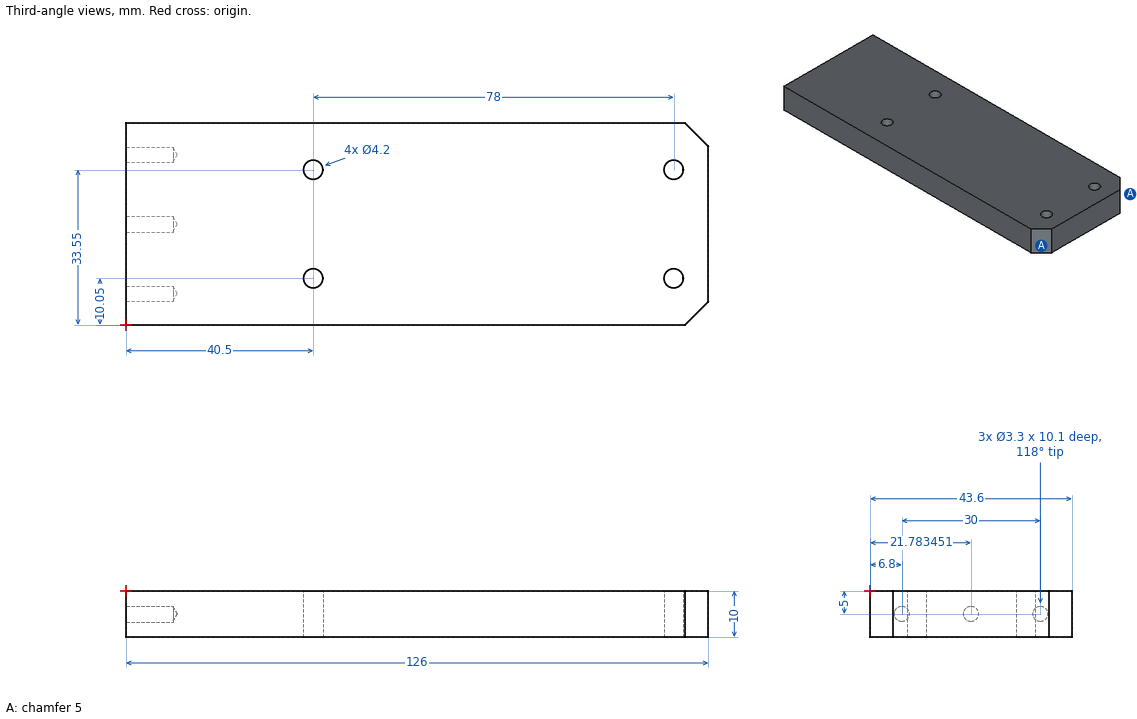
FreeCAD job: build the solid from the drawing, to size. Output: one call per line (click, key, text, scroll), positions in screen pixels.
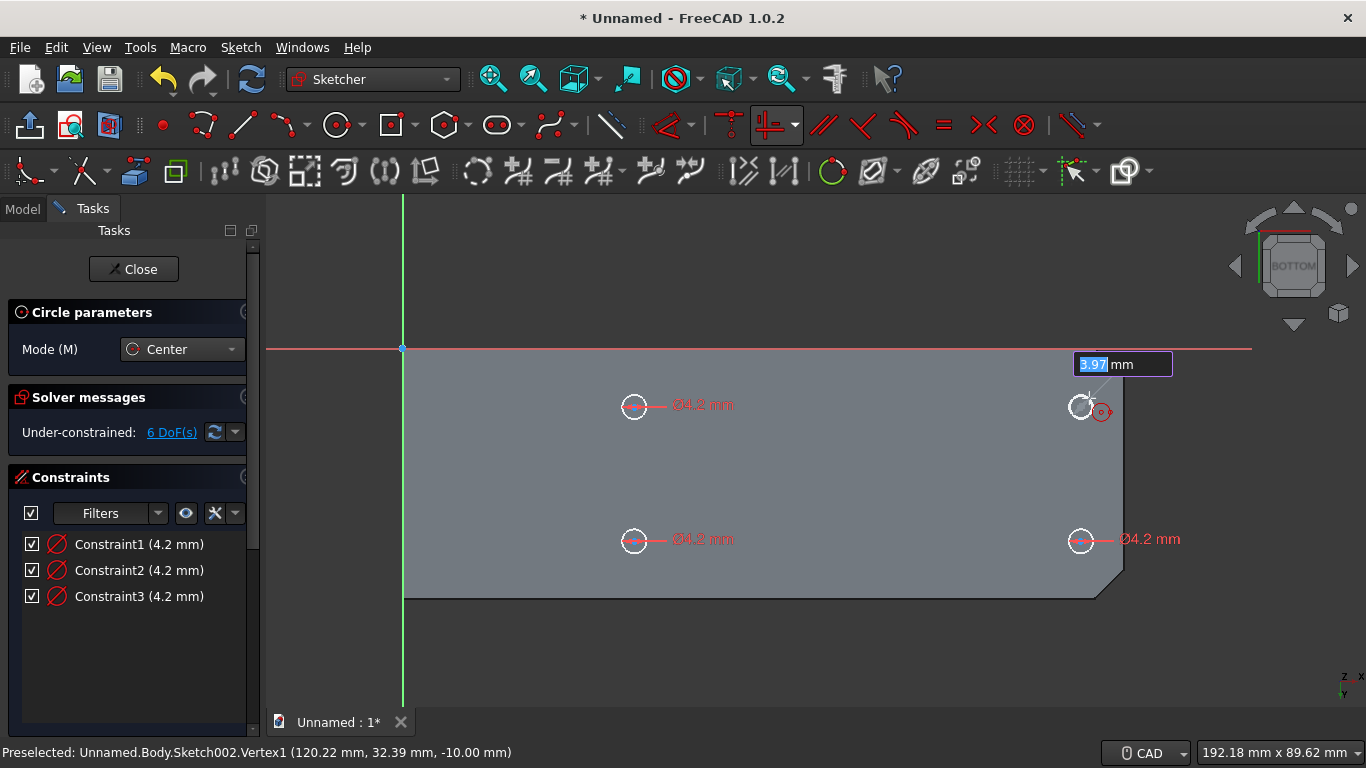
text(4.2)
key(Return)
key(Escape)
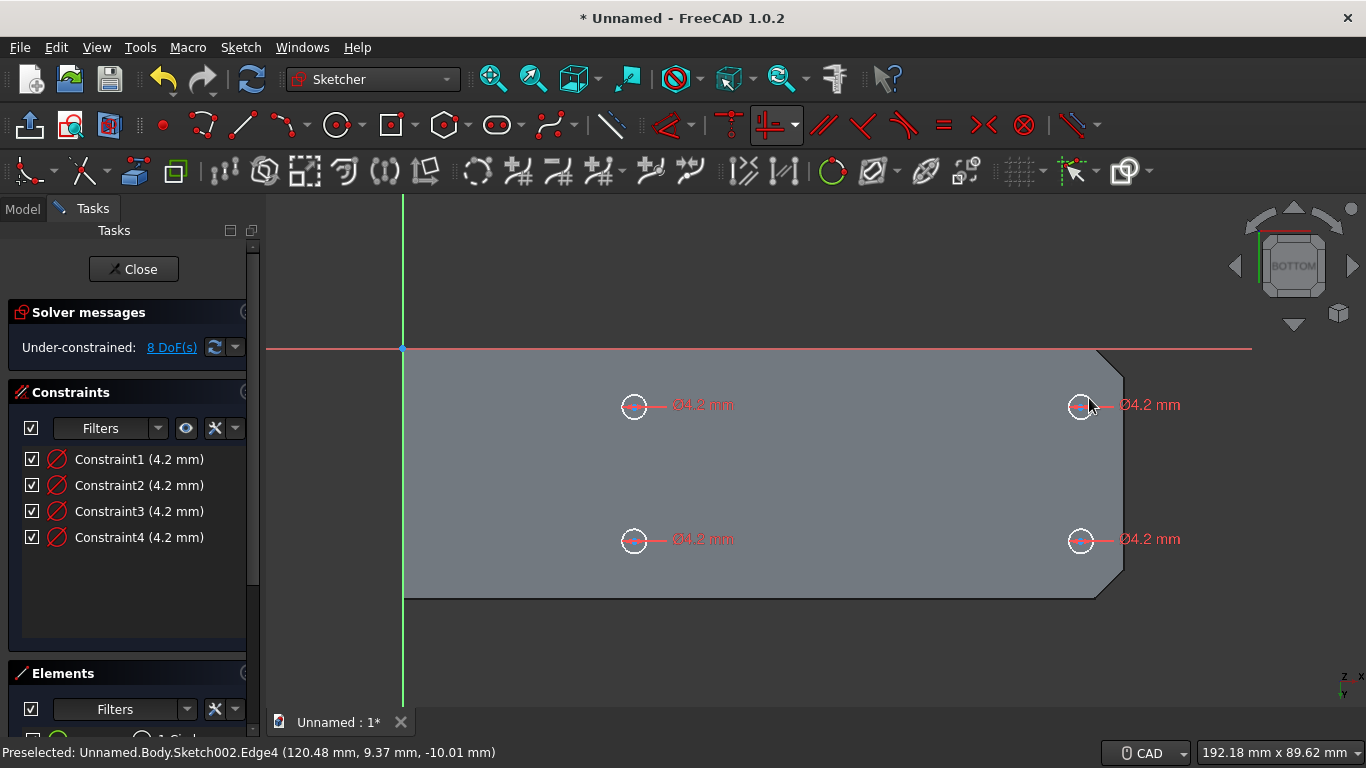
click(634, 541)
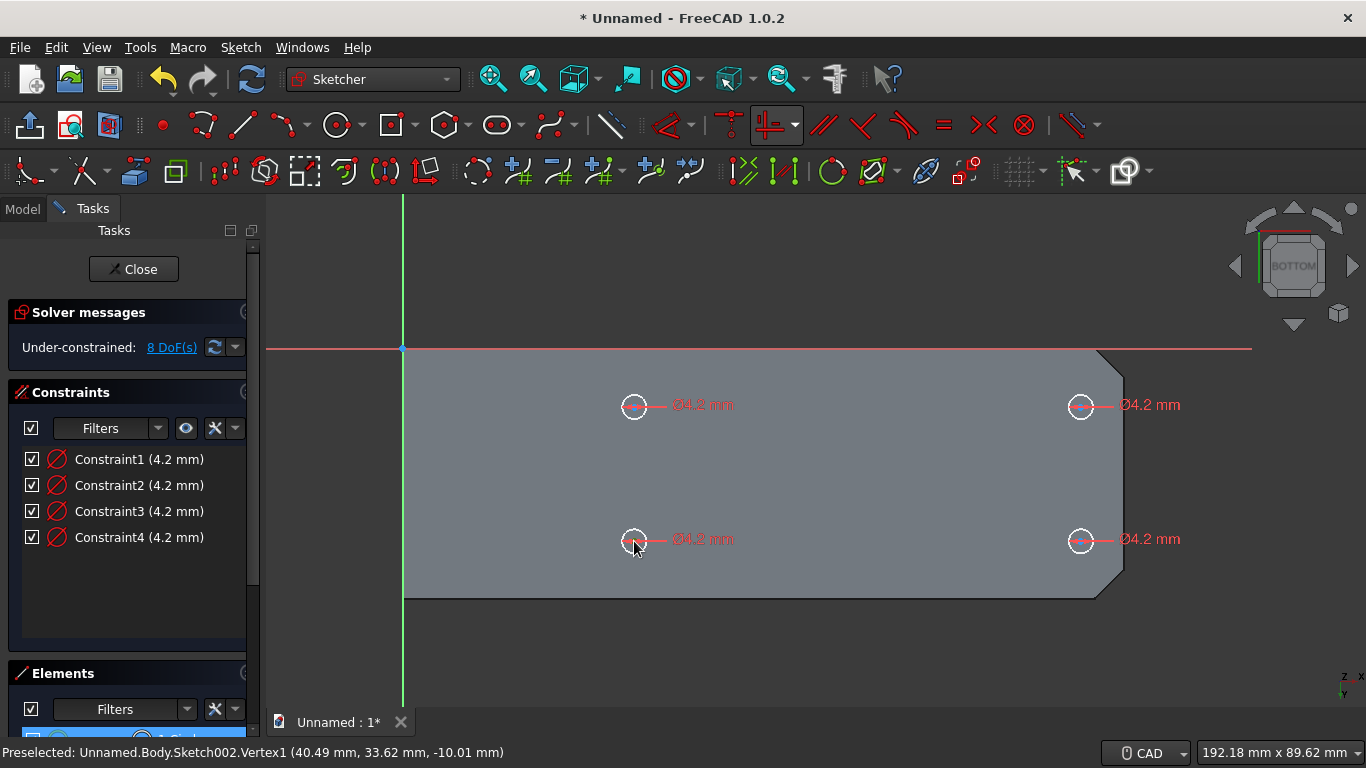
click(634, 407)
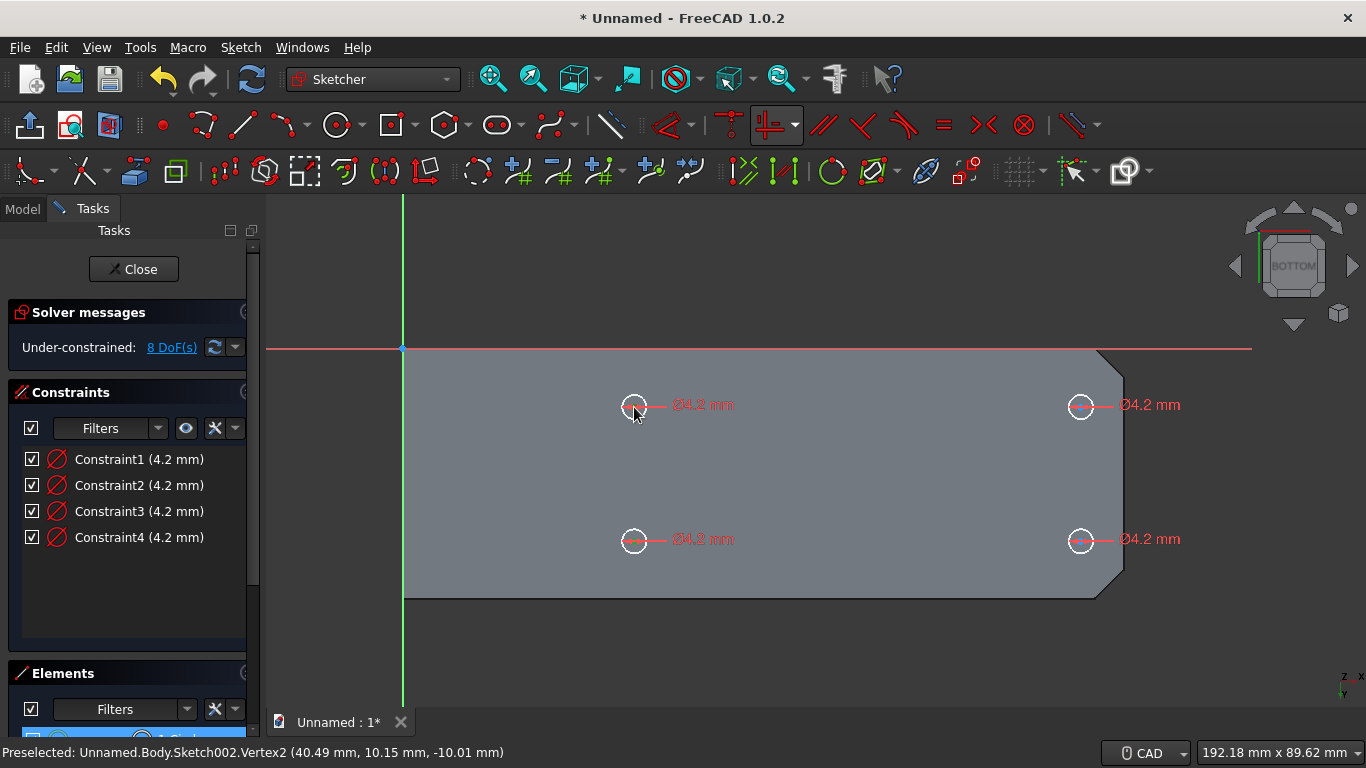
click(798, 126)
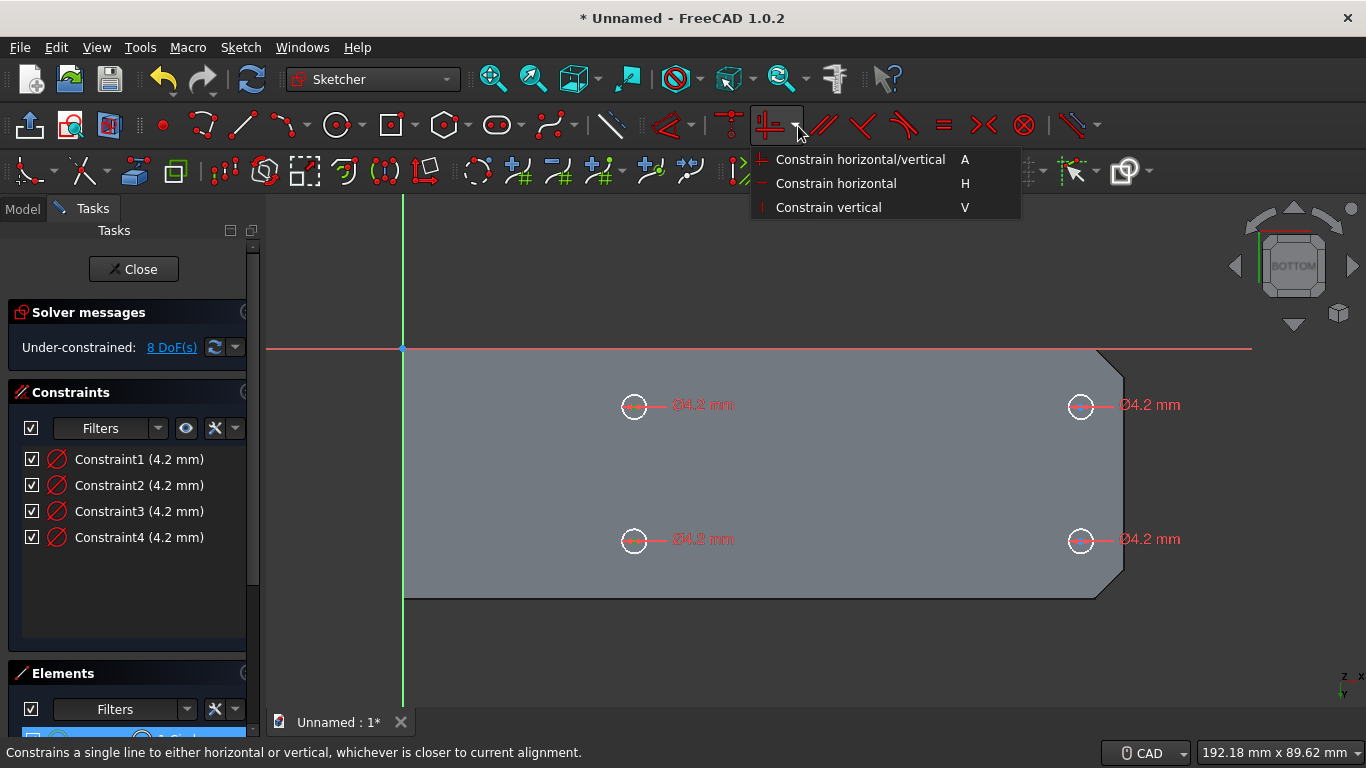
click(886, 207)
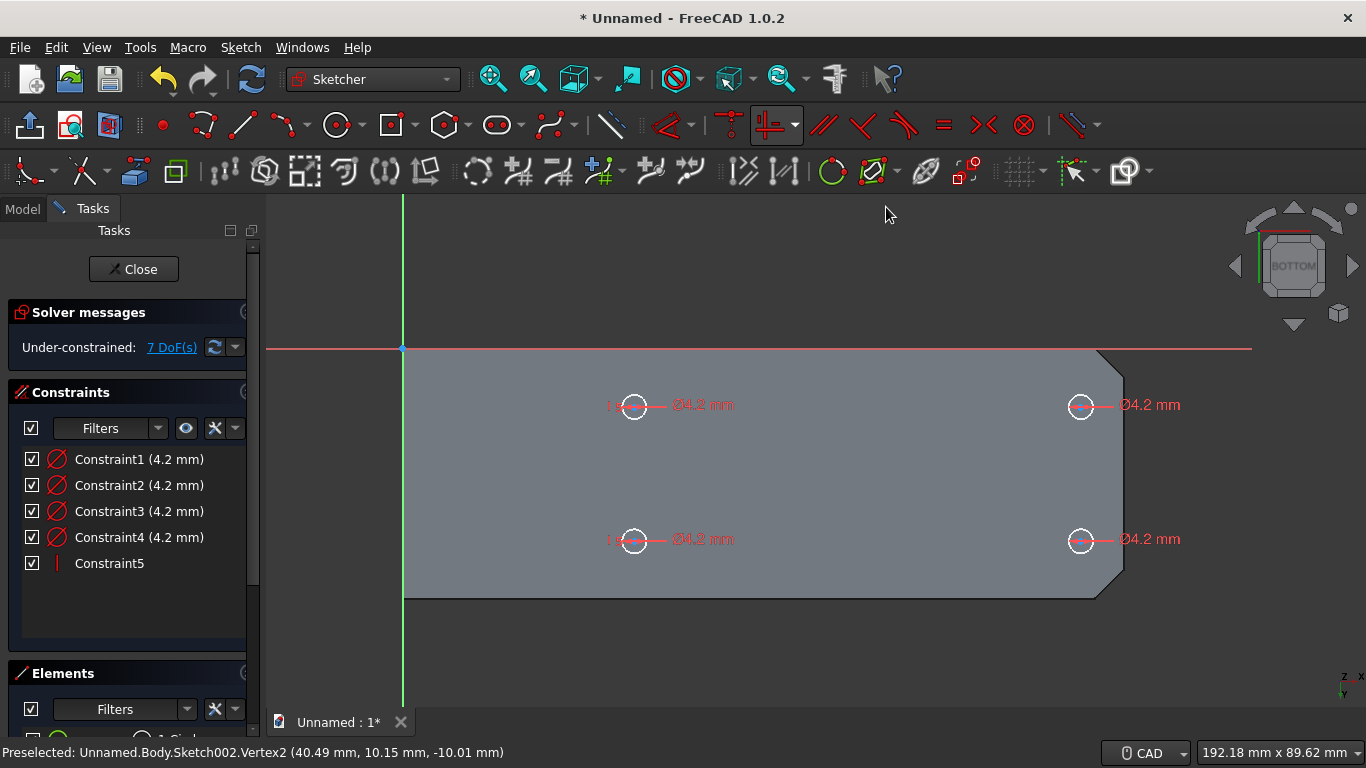
click(634, 541)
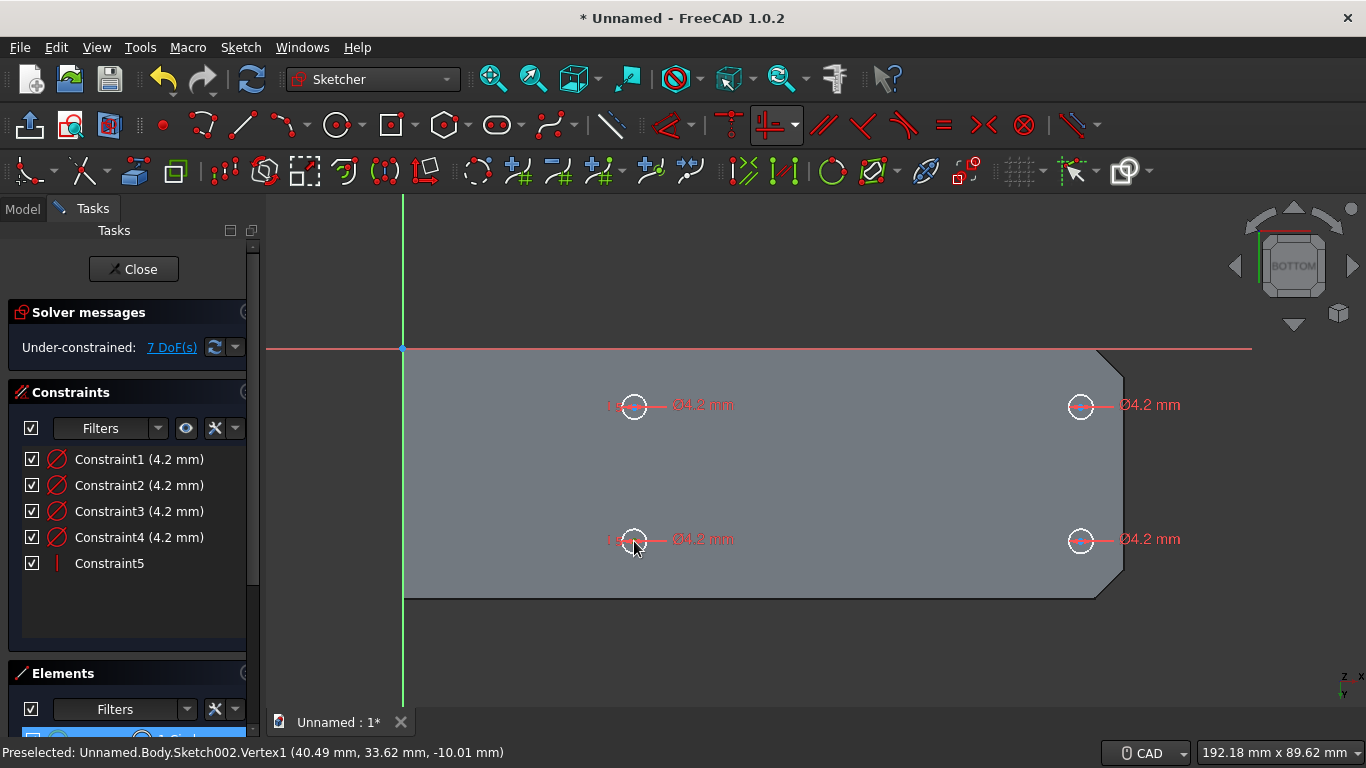
click(1081, 541)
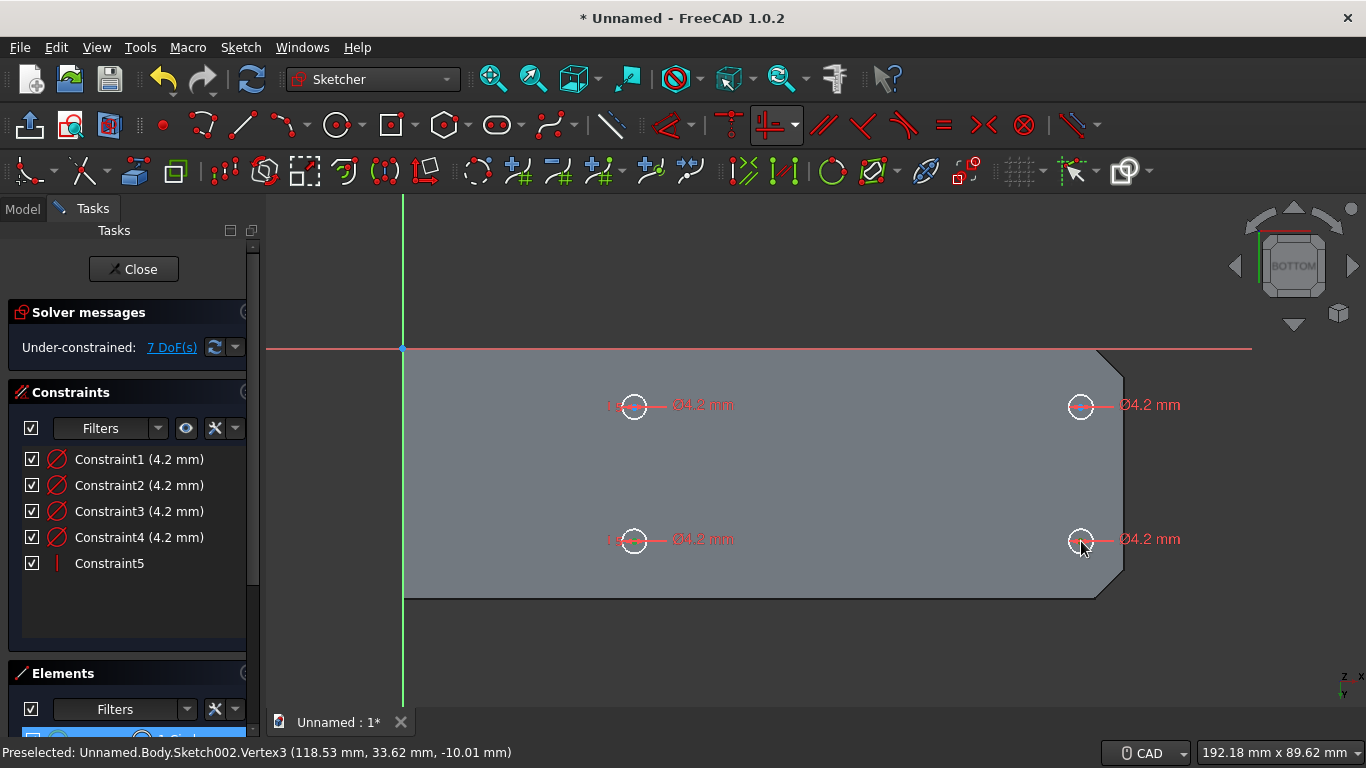
key(h)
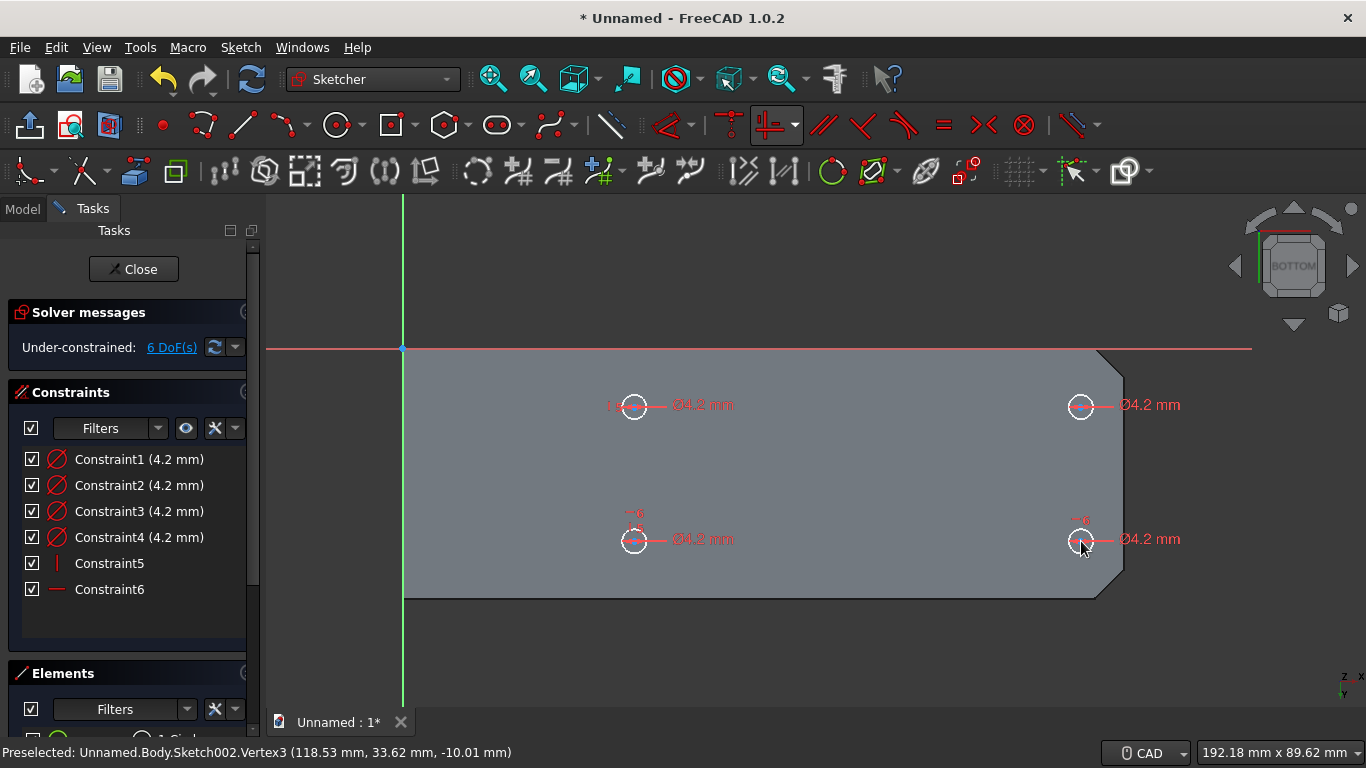
click(1081, 541)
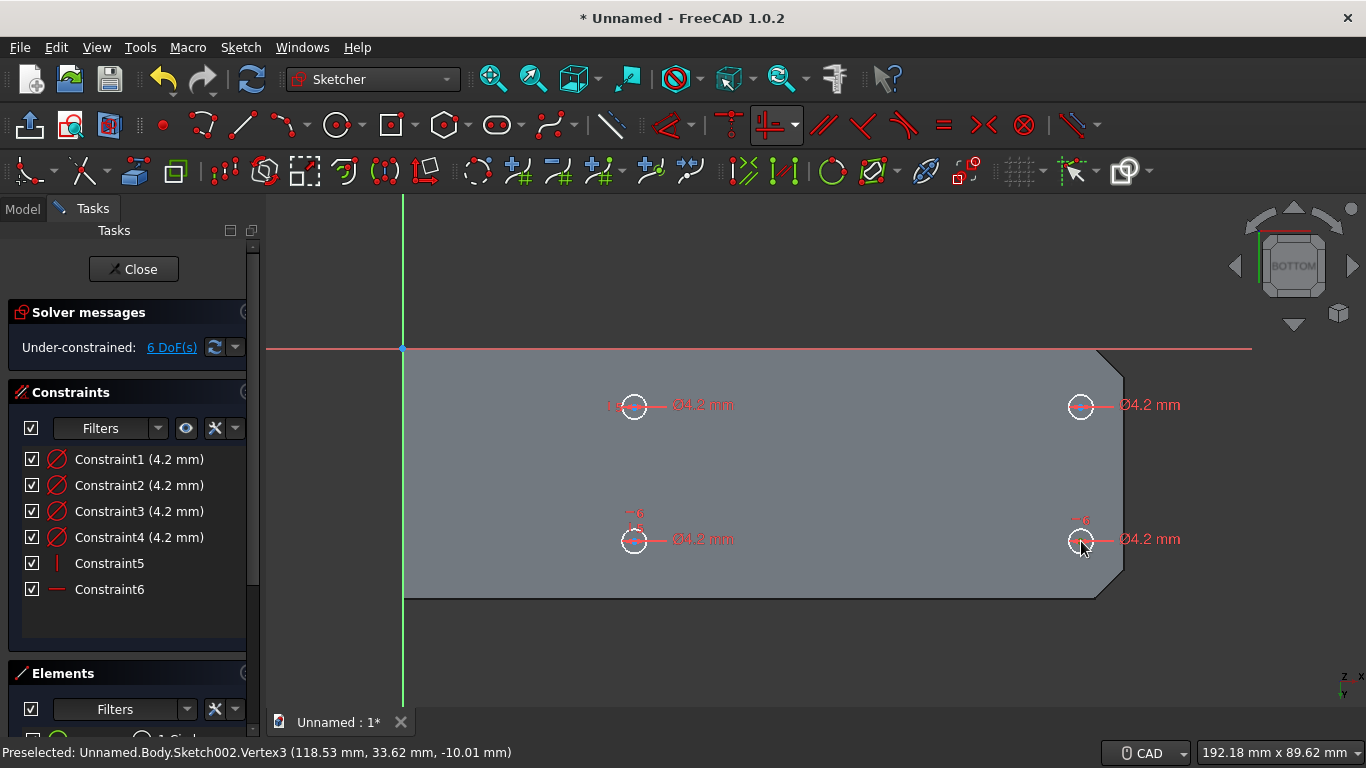
click(1081, 407)